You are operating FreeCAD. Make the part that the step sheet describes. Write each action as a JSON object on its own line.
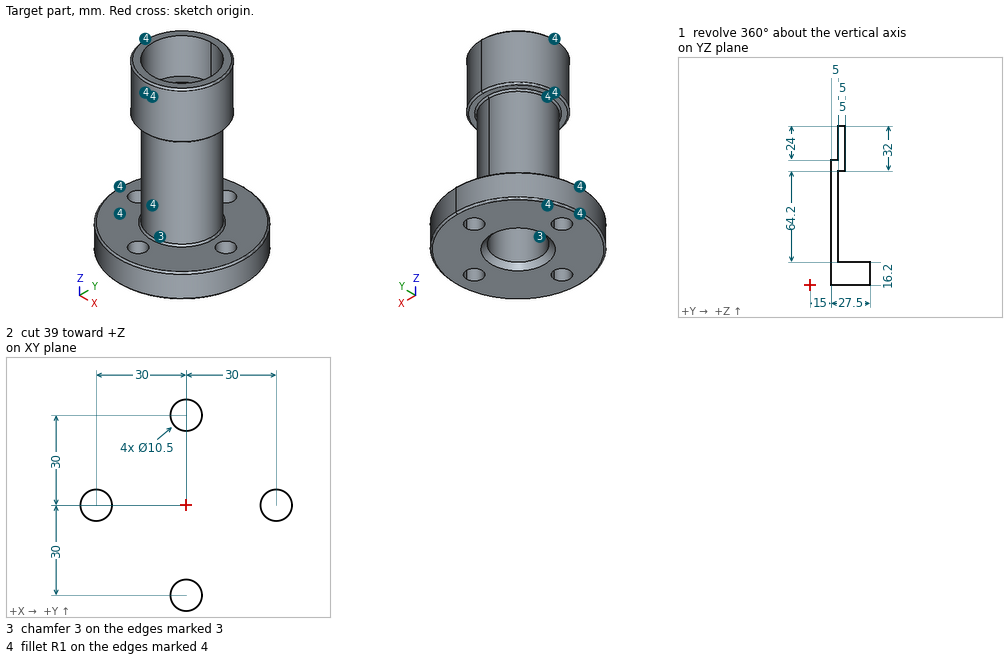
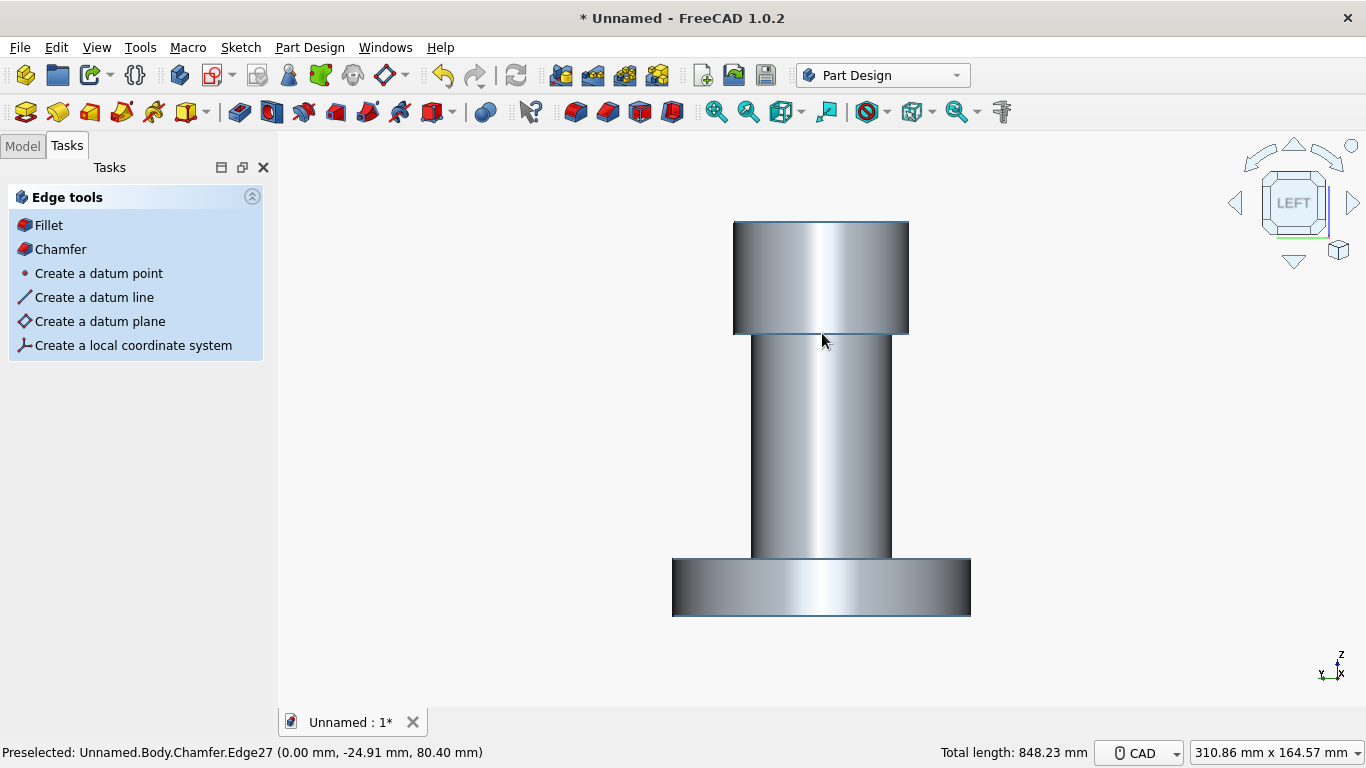
{"action": "key", "text": "v 3"}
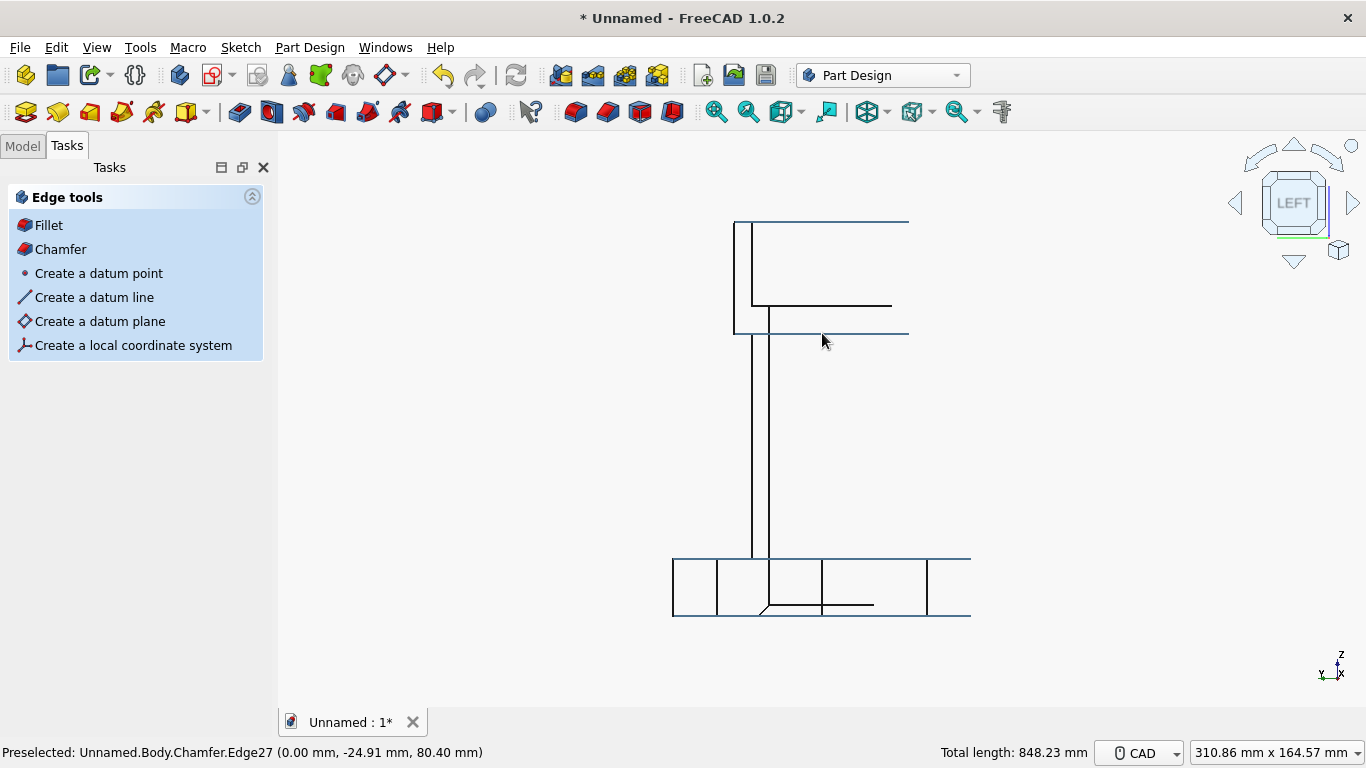
{"action": "key", "text": "0"}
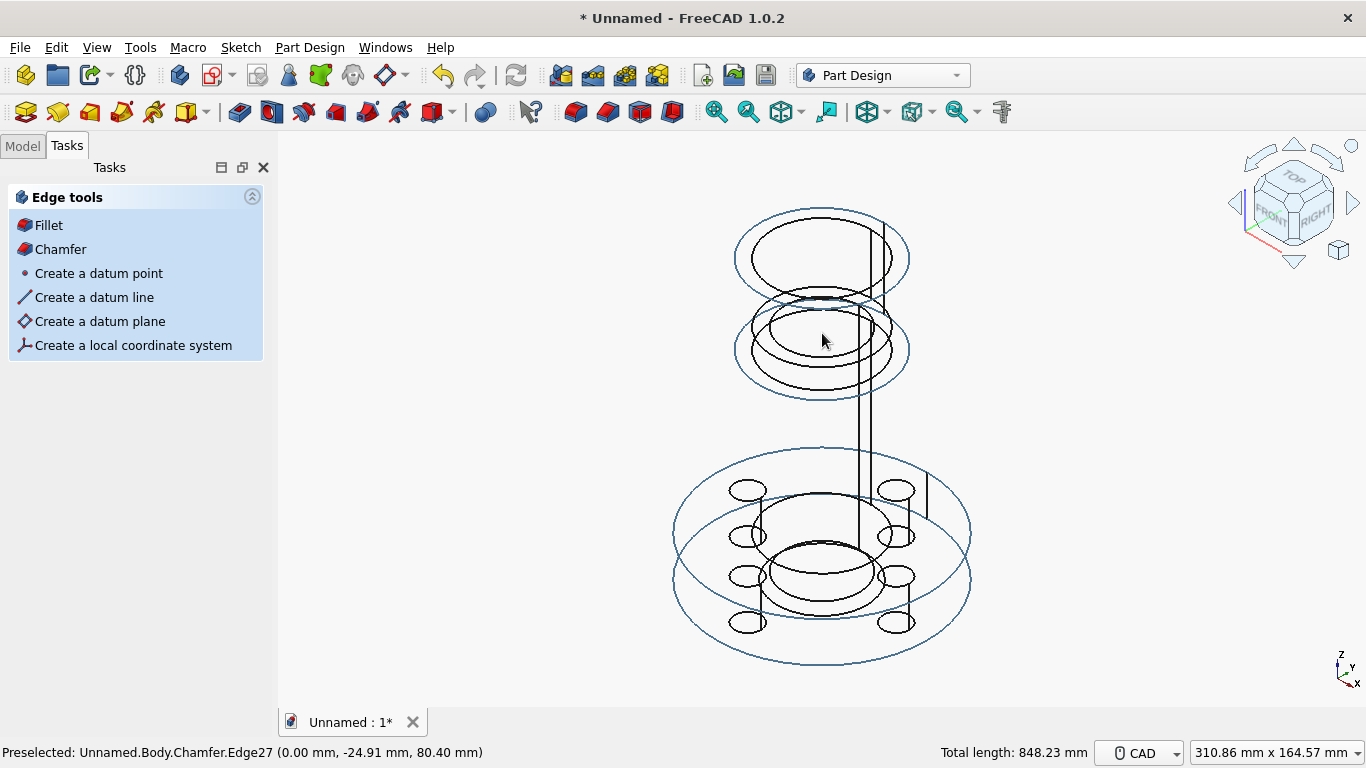
{"action": "left_click", "coordinate": [773, 377], "text": "ctrl"}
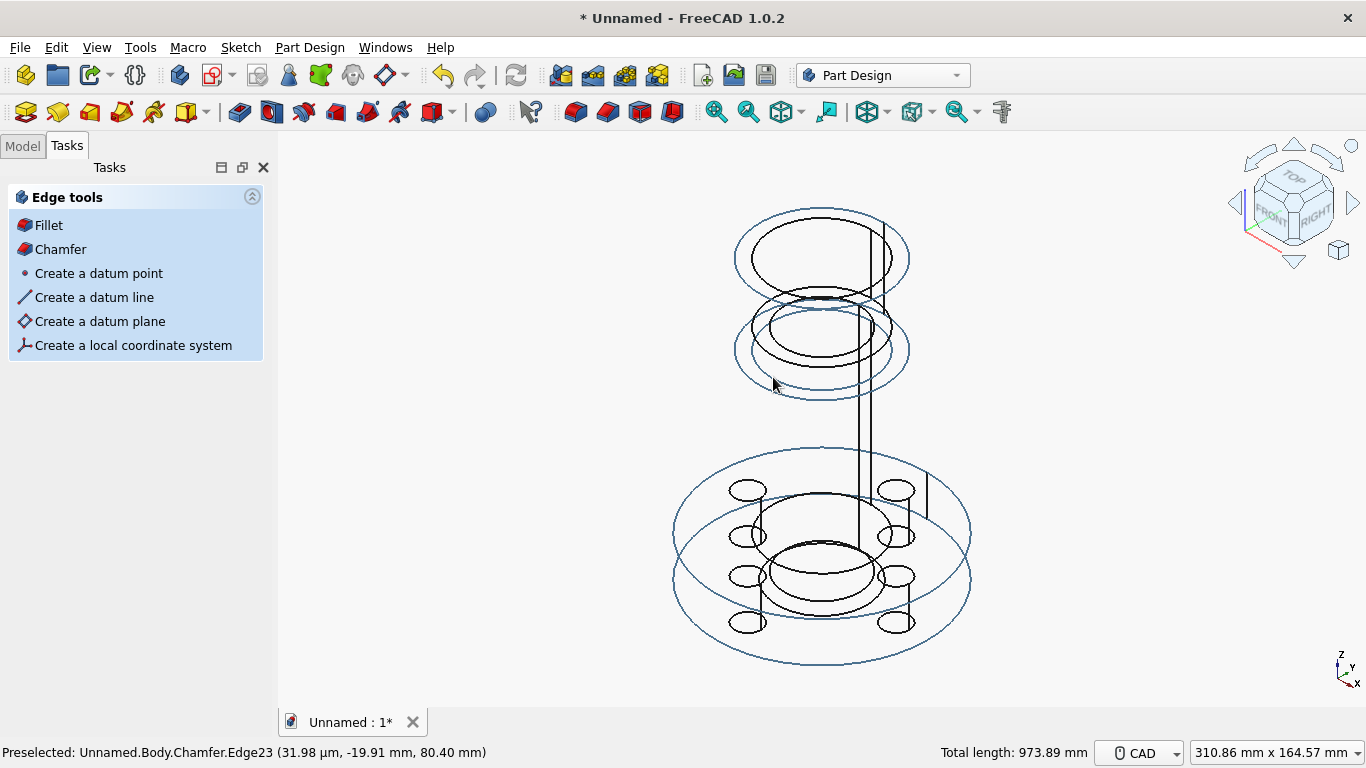
{"action": "left_click", "coordinate": [773, 561], "text": "ctrl"}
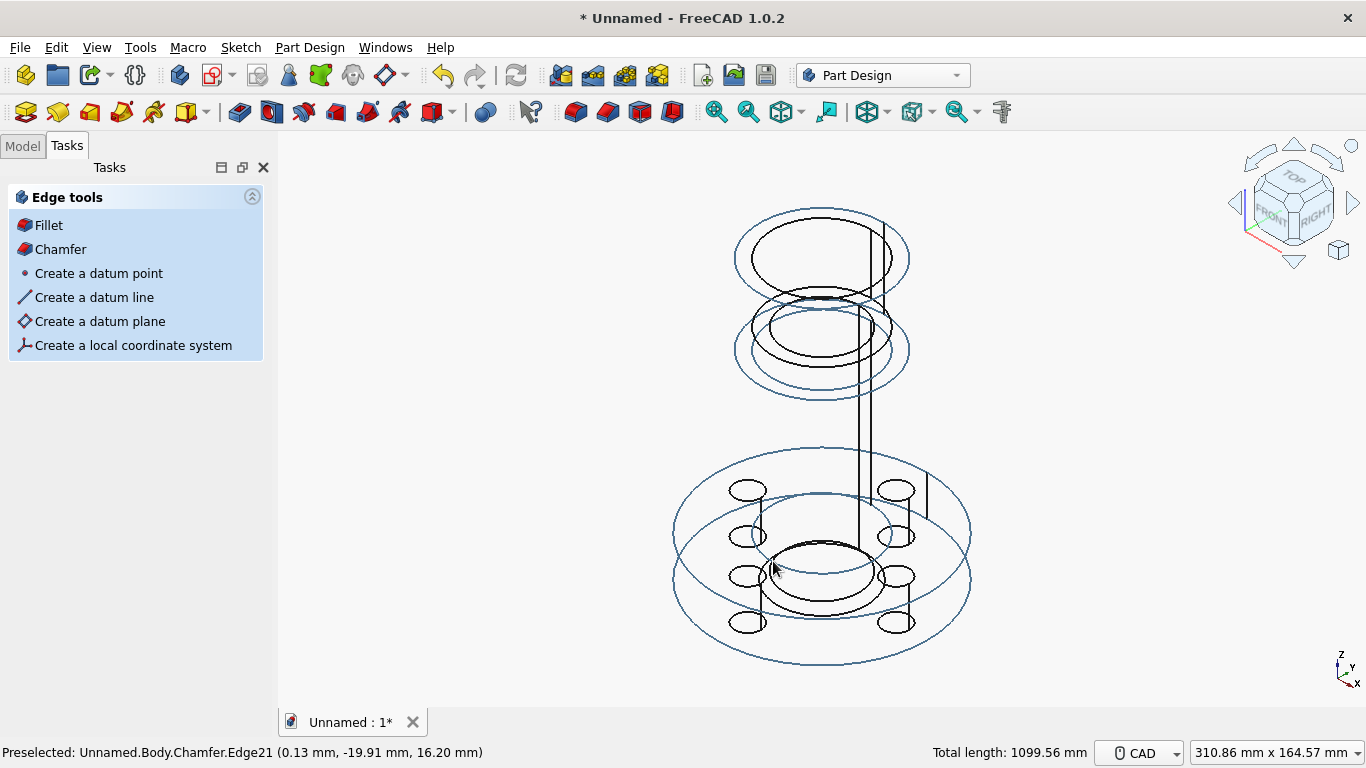
{"action": "key", "text": "v 1"}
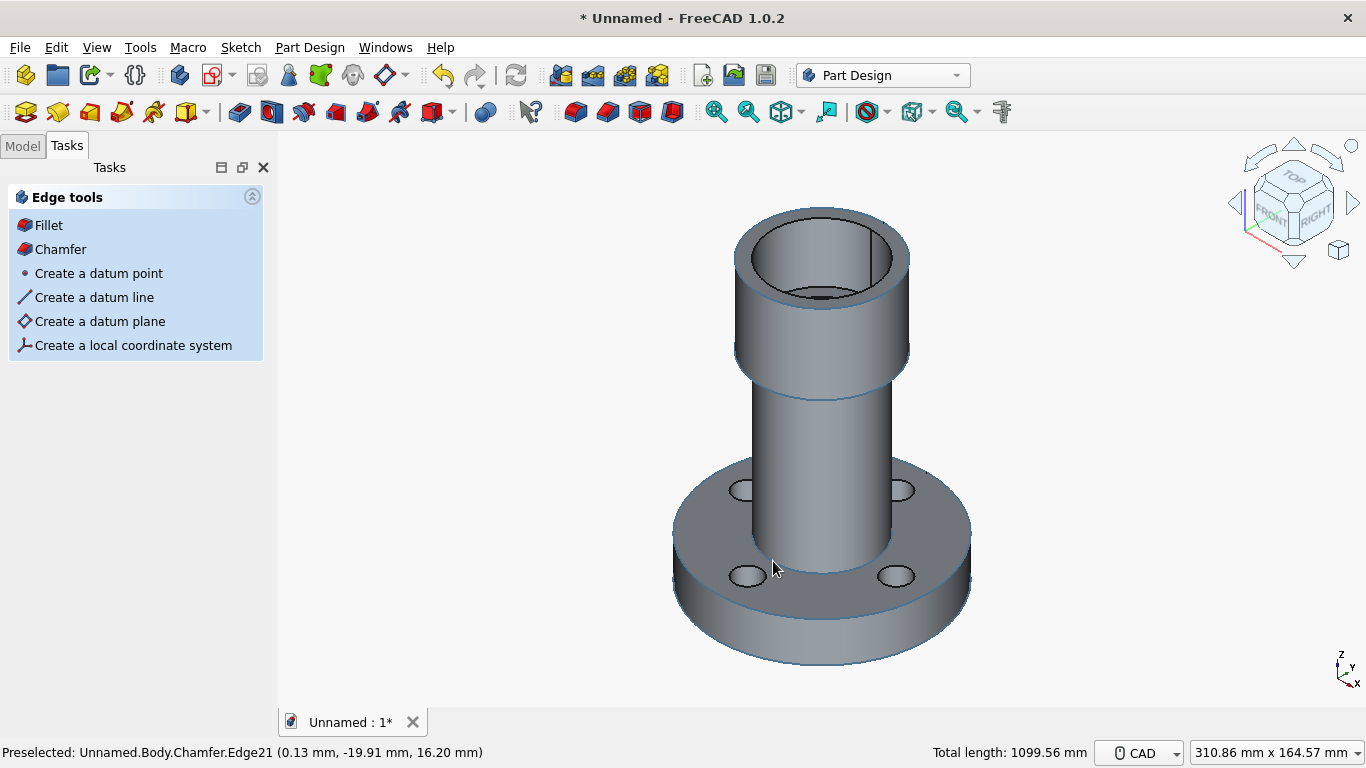
{"action": "left_click", "coordinate": [576, 112]}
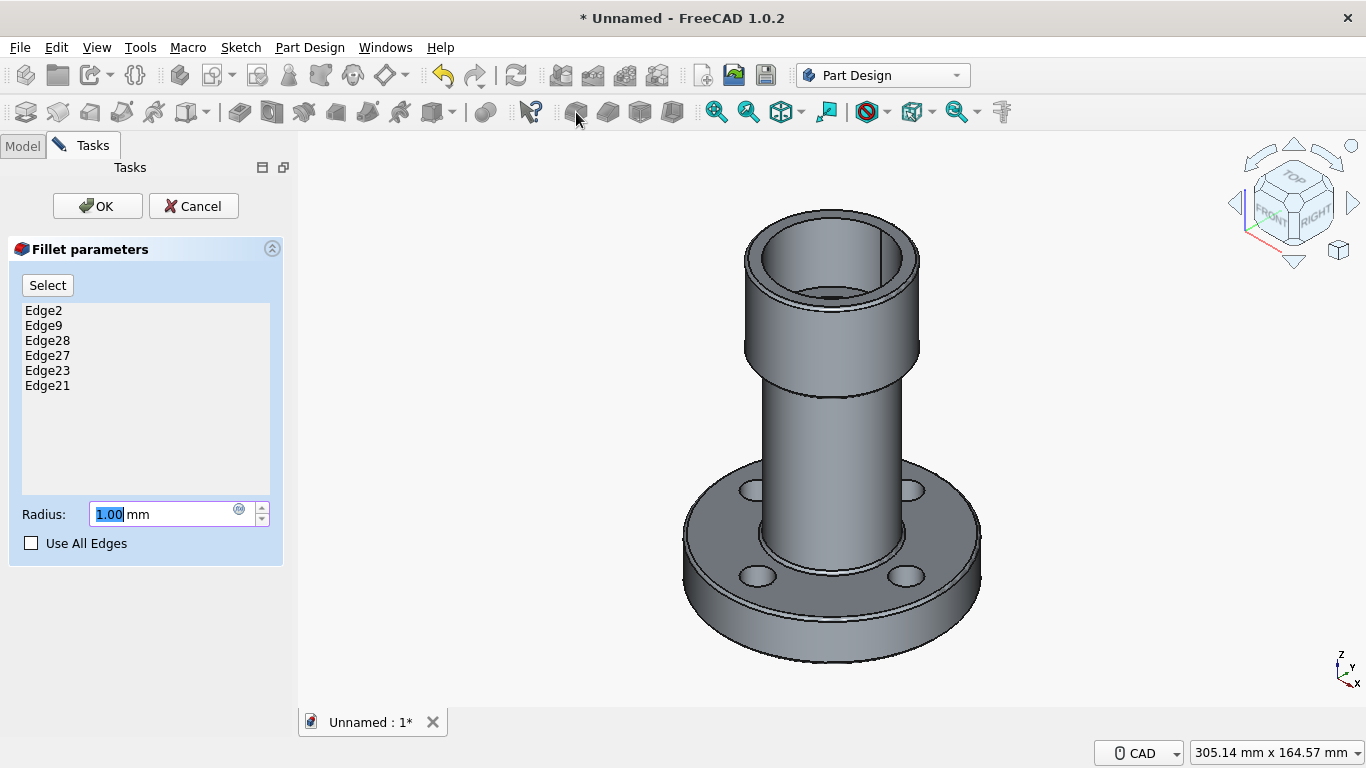
{"action": "type", "text": "1"}
{"action": "key", "text": "Tab"}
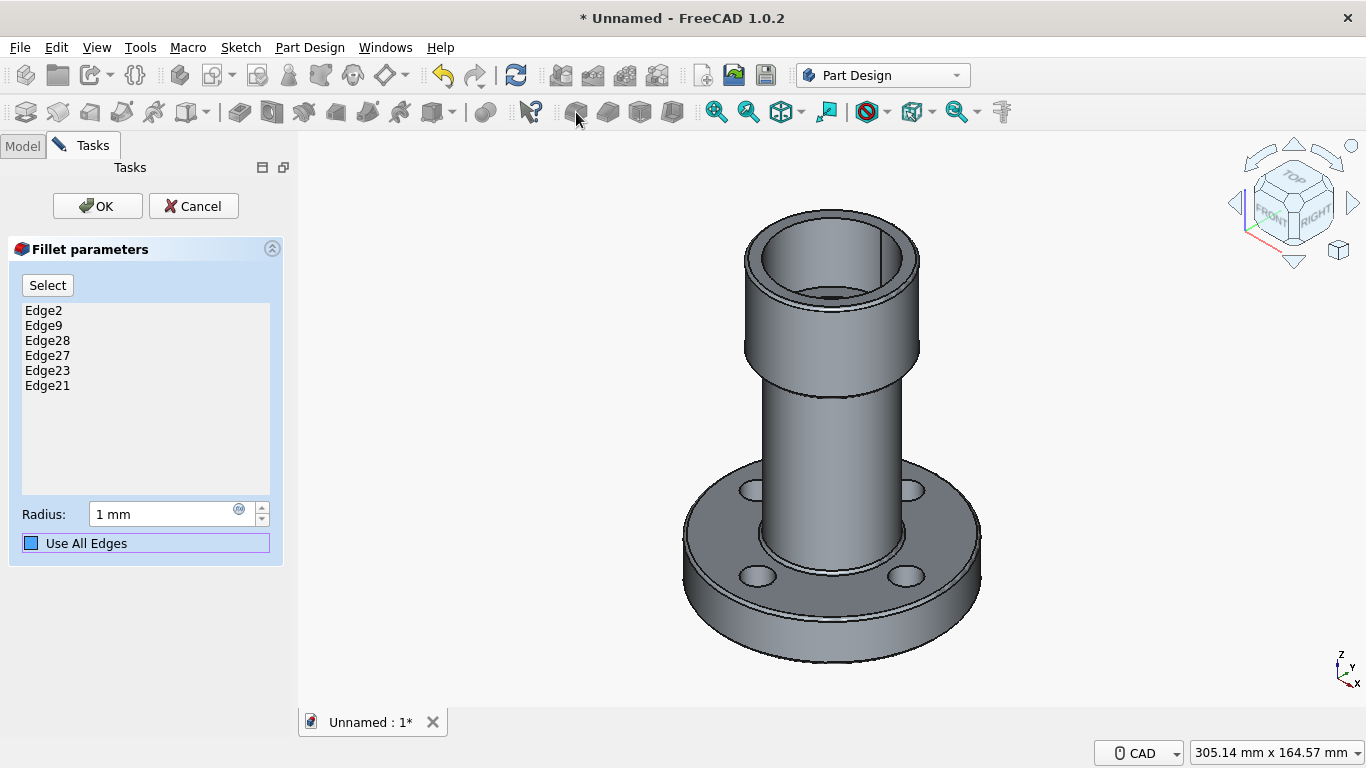
{"action": "left_click", "coordinate": [98, 206]}